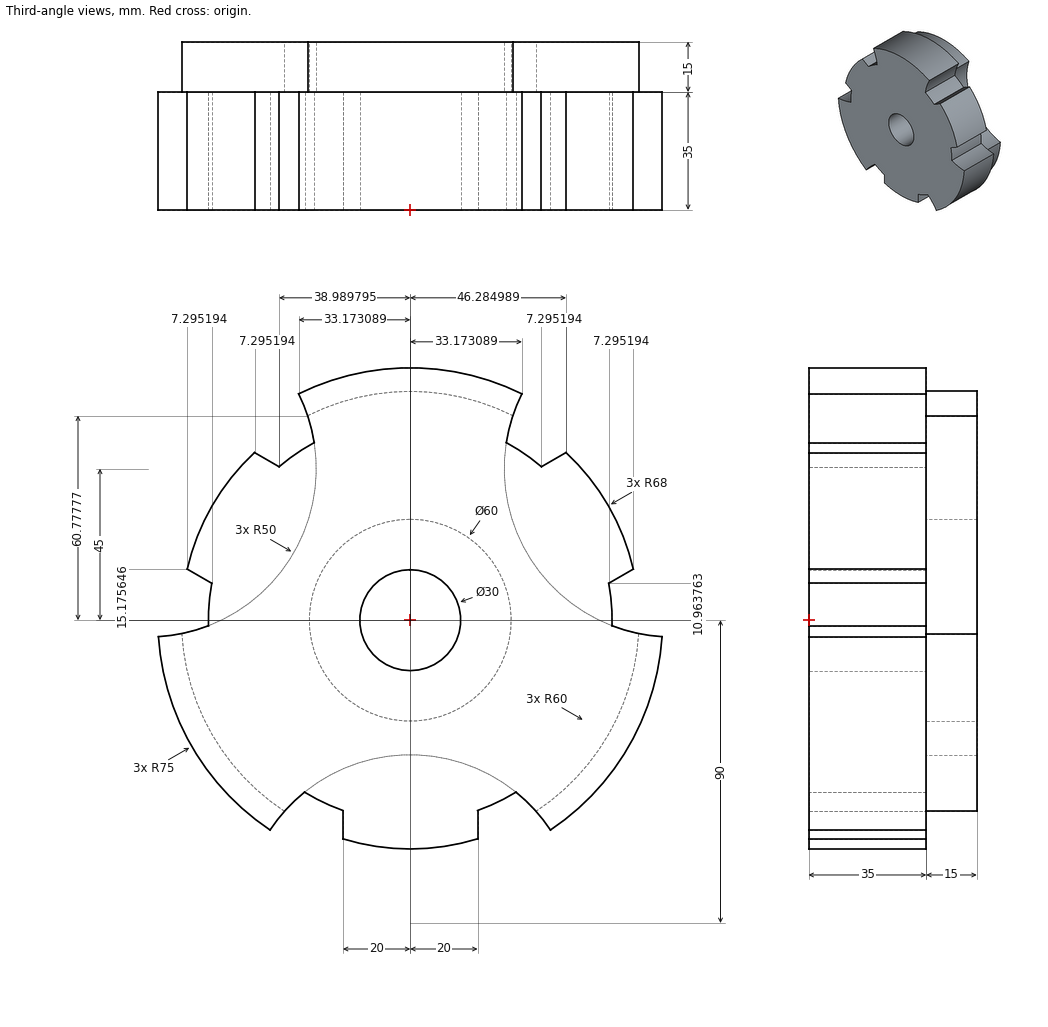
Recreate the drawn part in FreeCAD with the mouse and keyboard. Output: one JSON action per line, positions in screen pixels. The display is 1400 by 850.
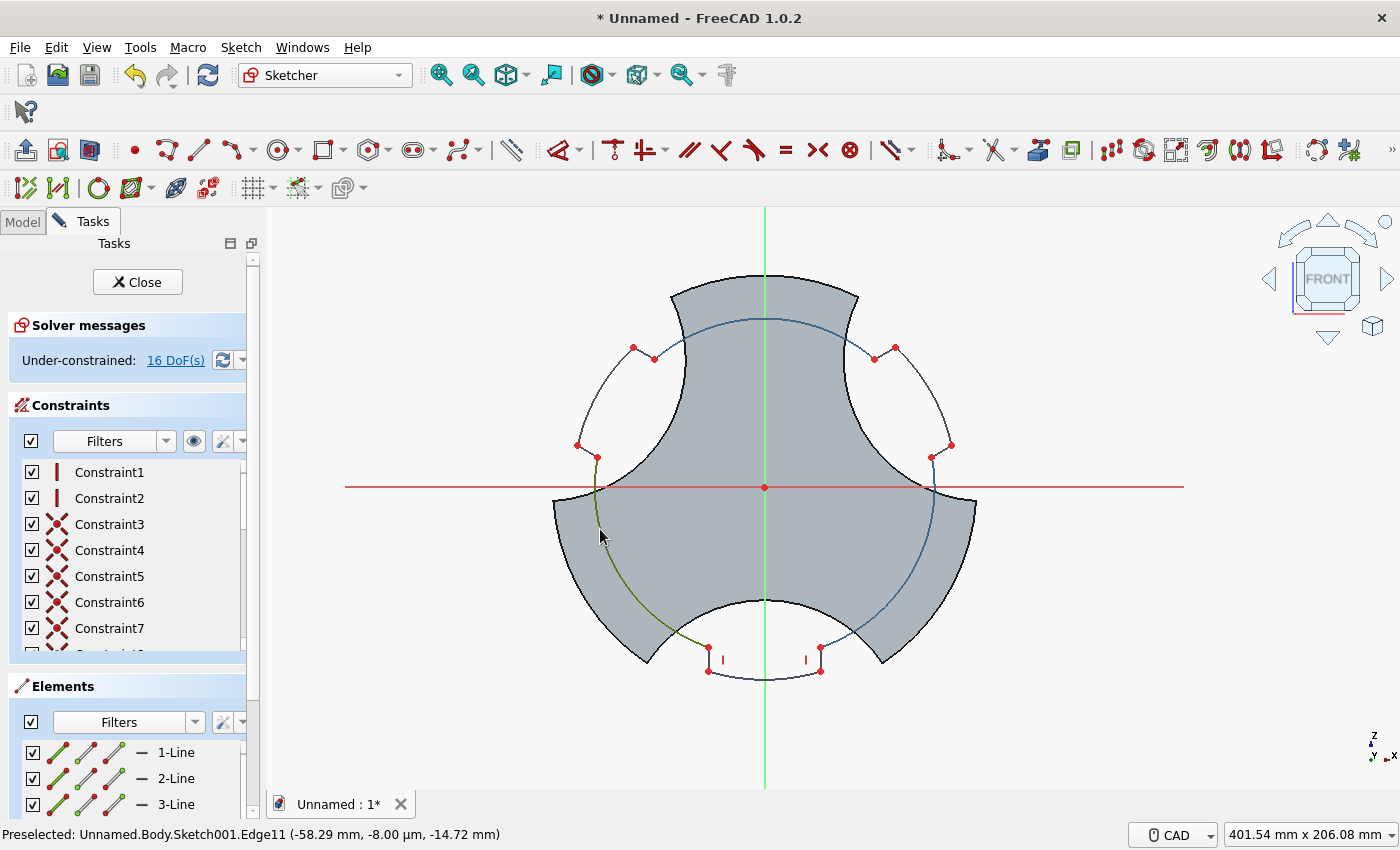
{"action": "key", "text": "e"}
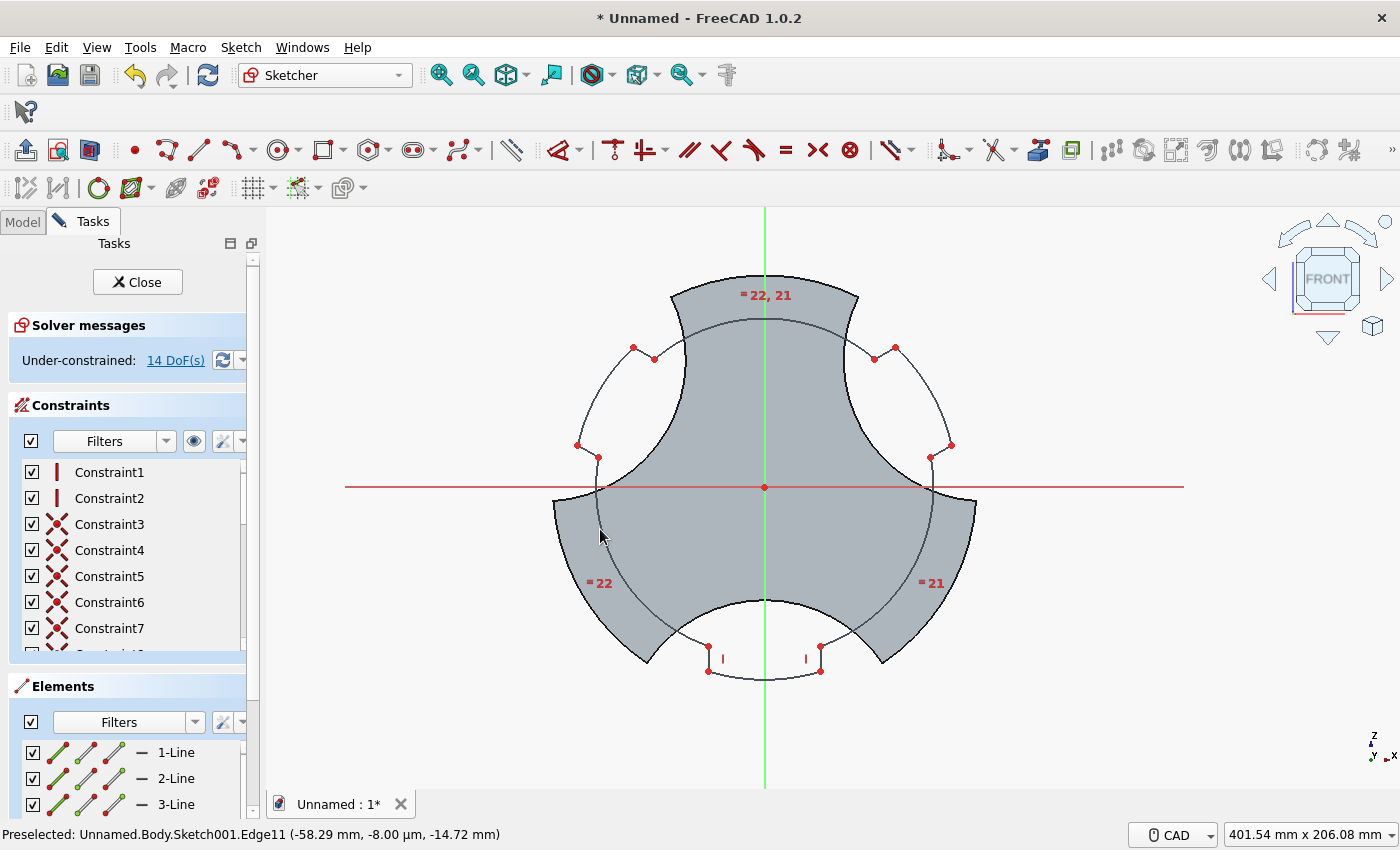
{"action": "left_click", "coordinate": [941, 413]}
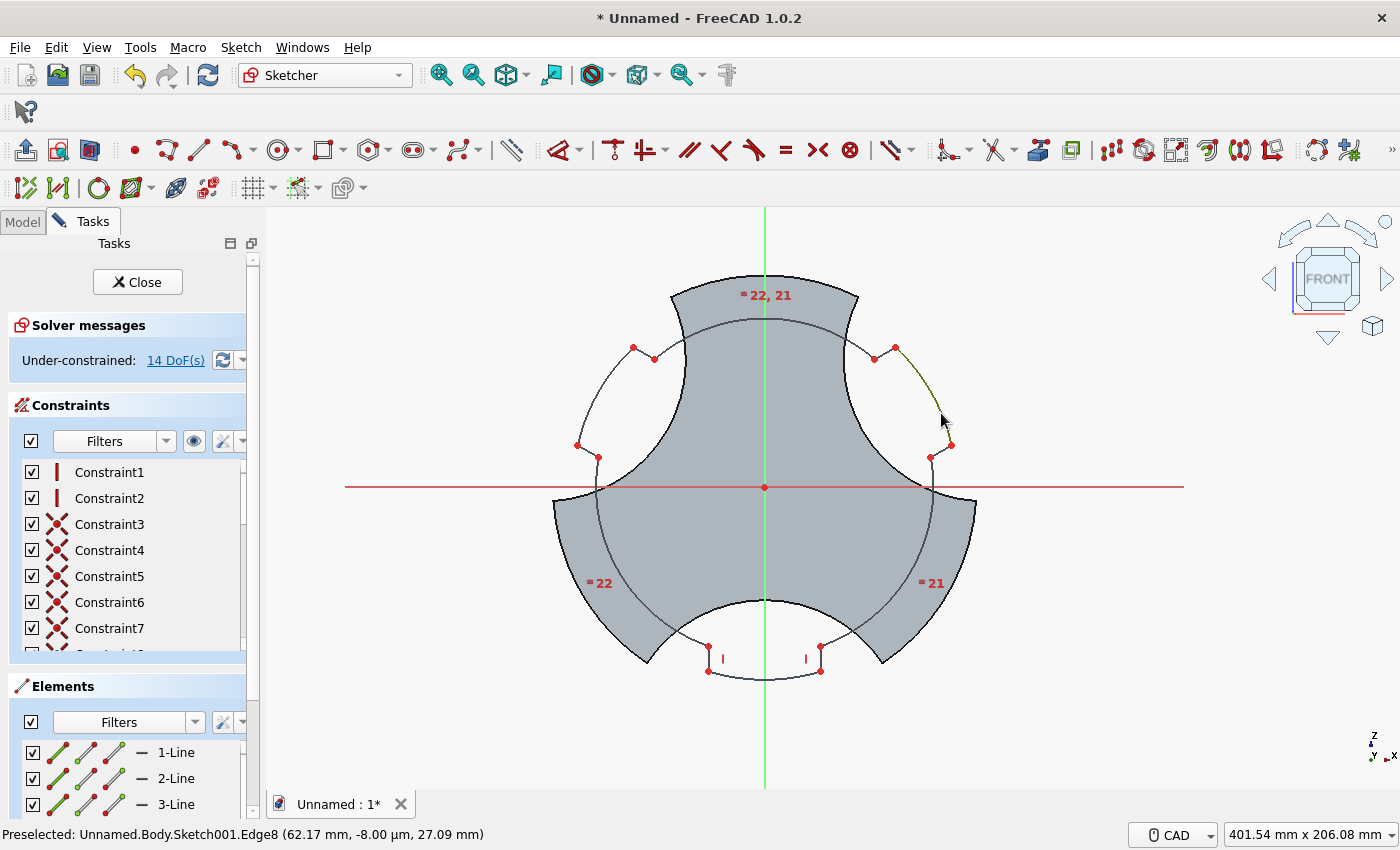
{"action": "left_click", "coordinate": [611, 373]}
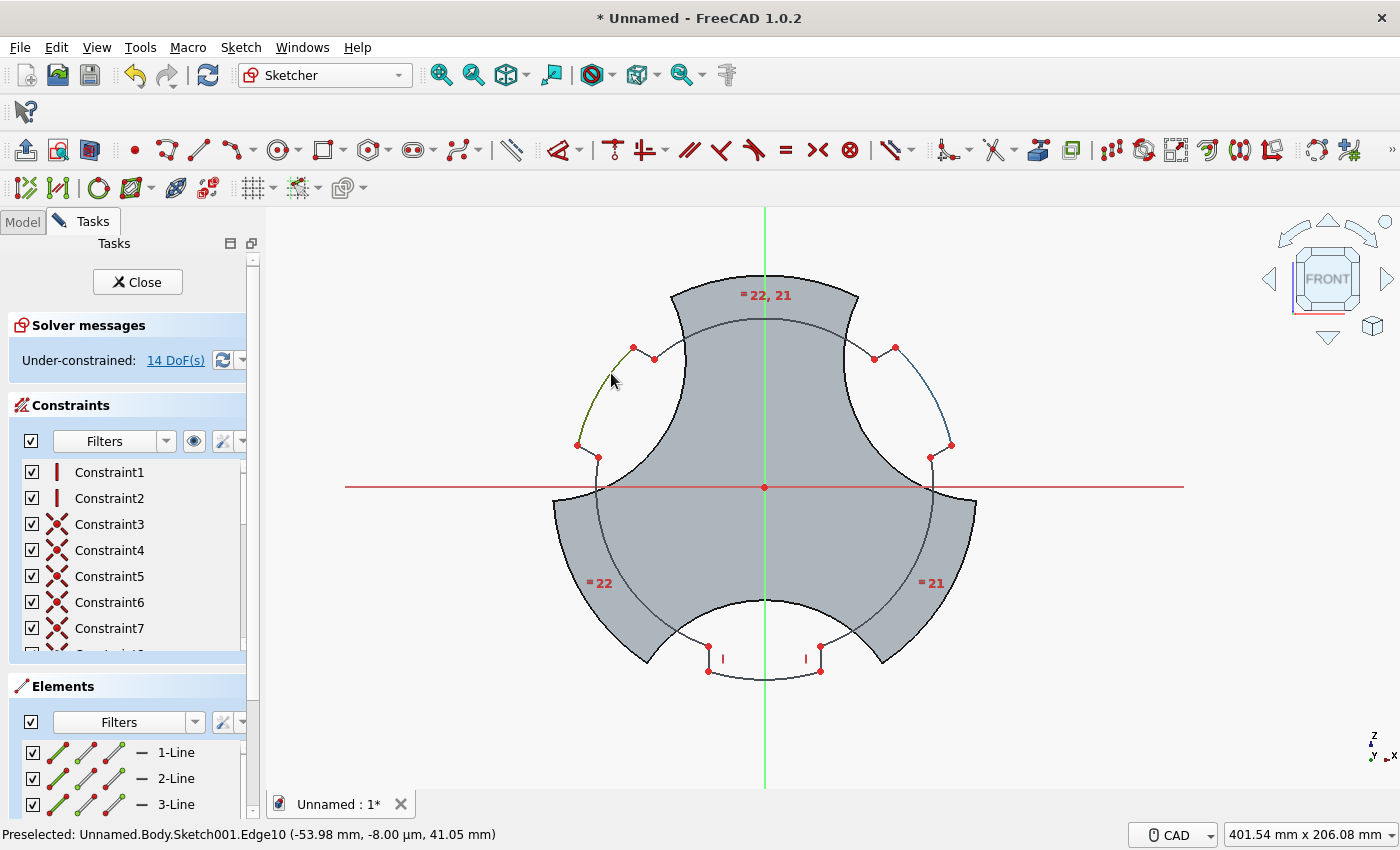
{"action": "left_click", "coordinate": [742, 678]}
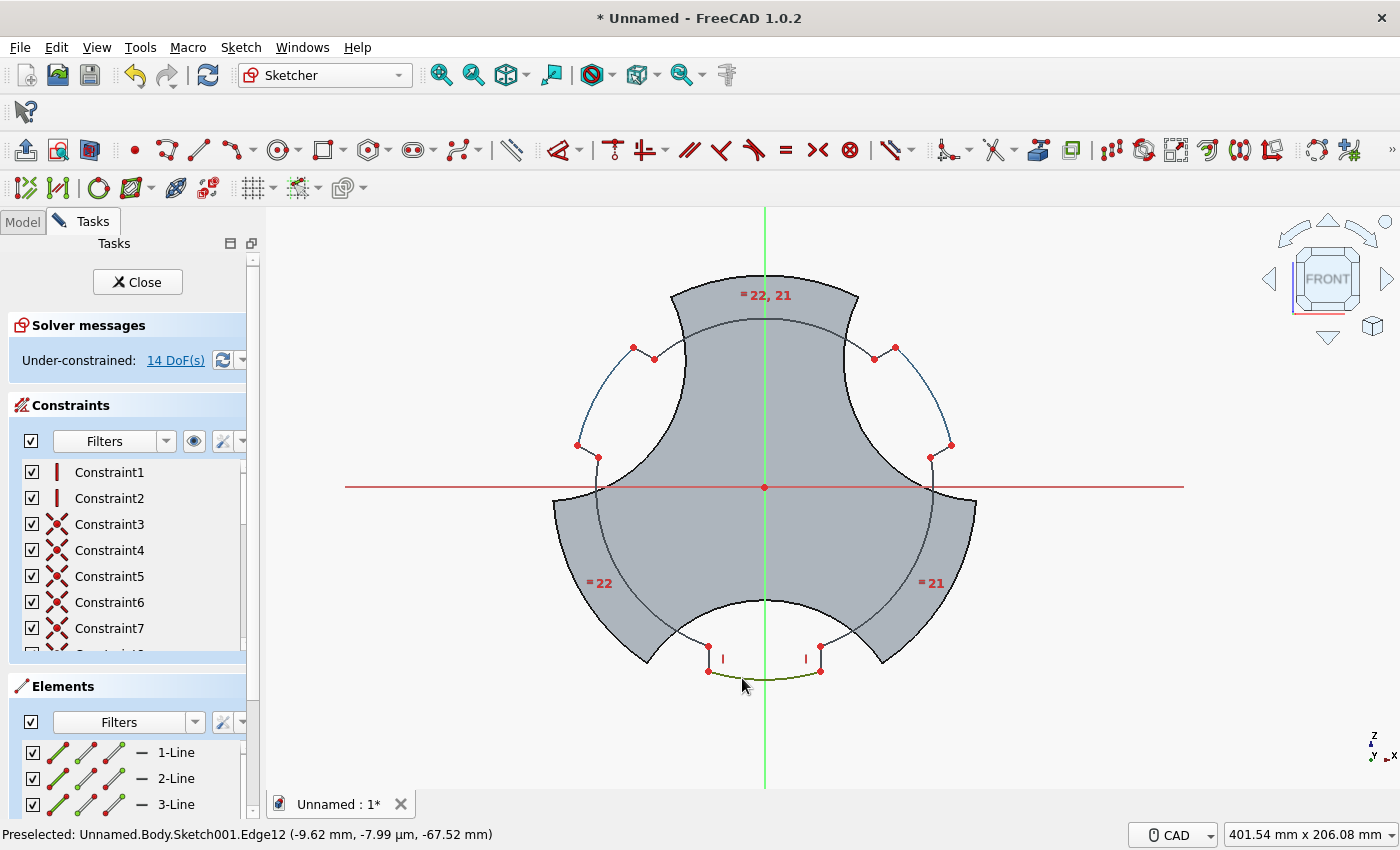
{"action": "left_click", "coordinate": [786, 150]}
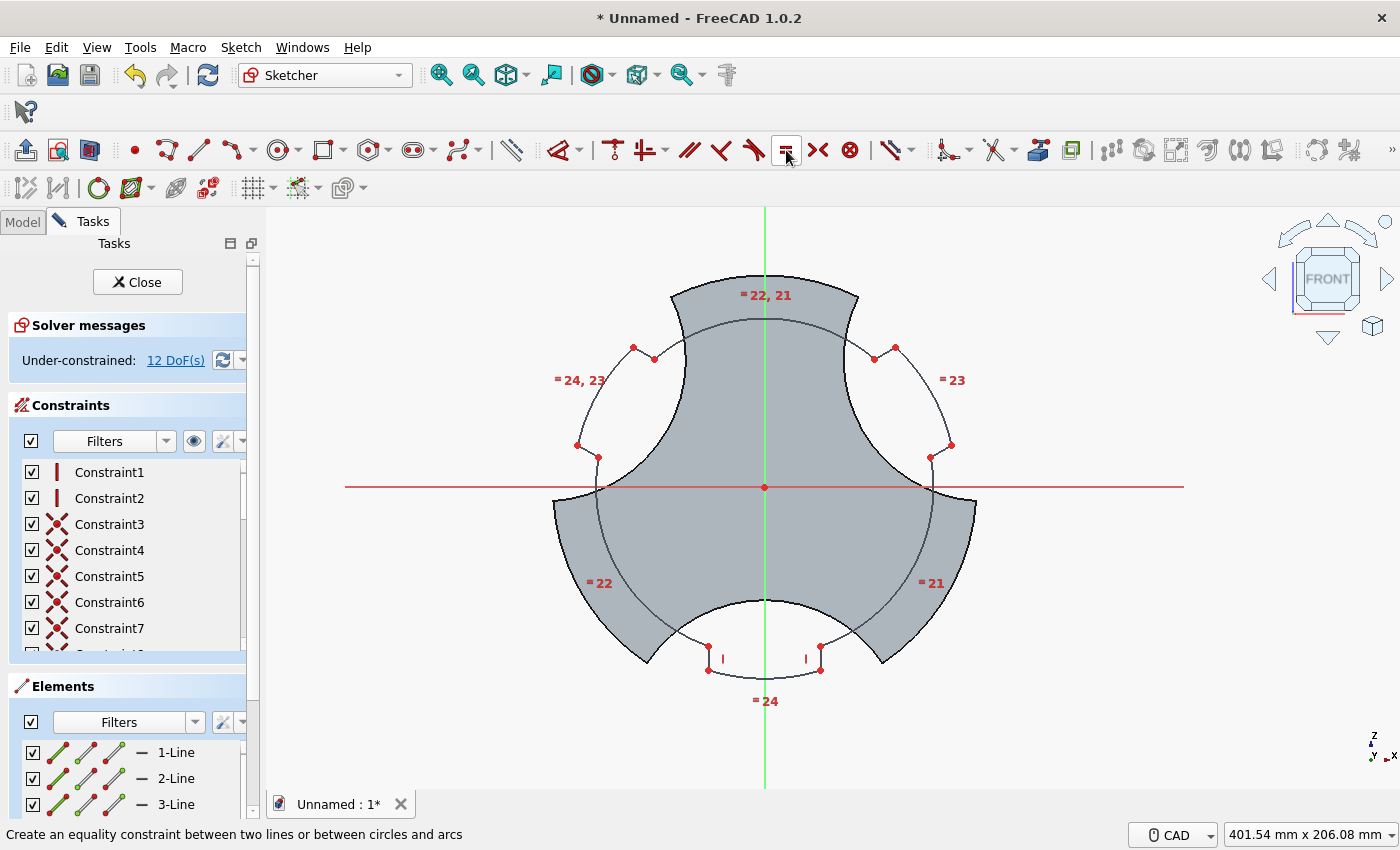
{"action": "left_click", "coordinate": [558, 150]}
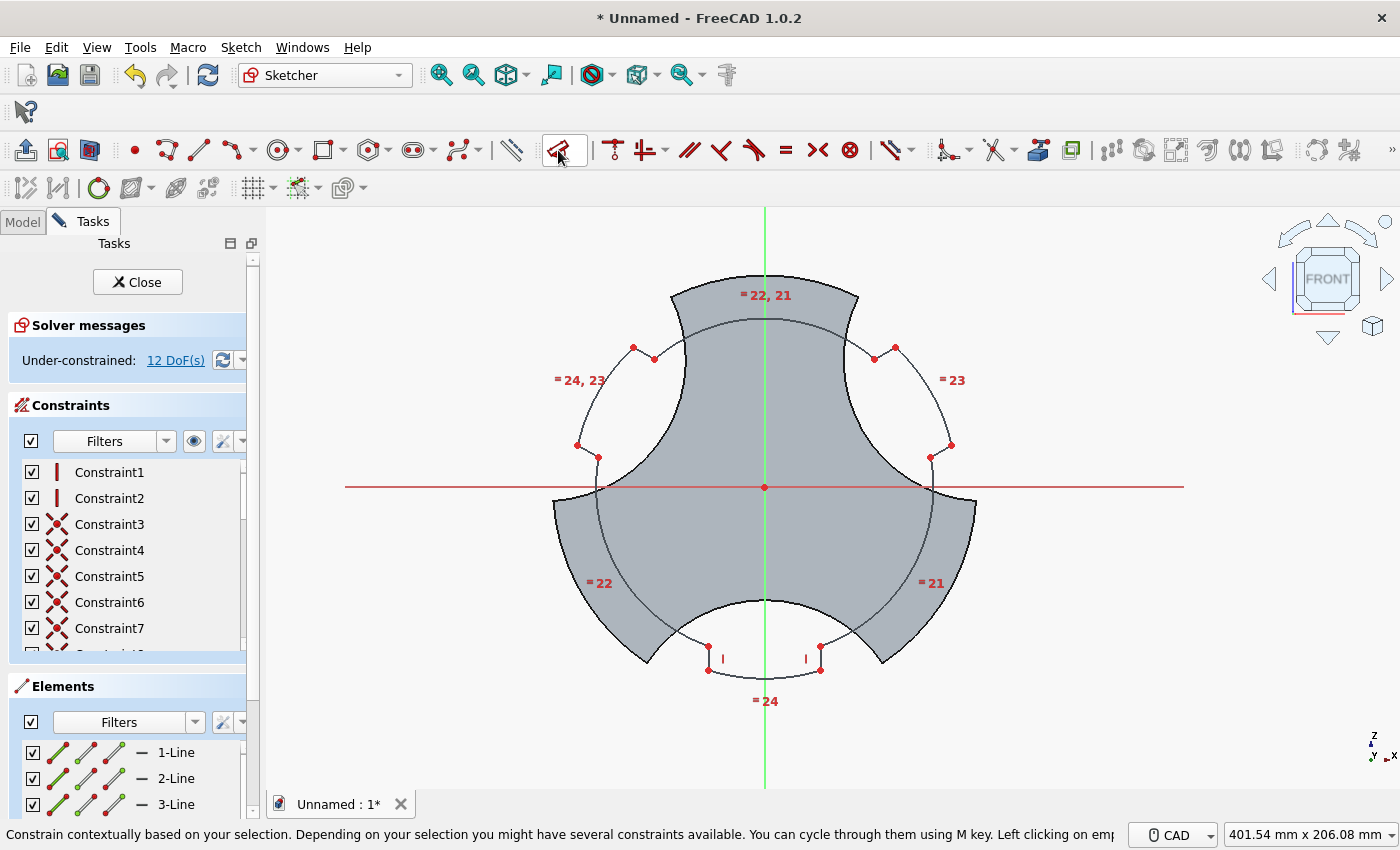
{"action": "left_click", "coordinate": [881, 609]}
{"action": "left_click", "coordinate": [903, 632]}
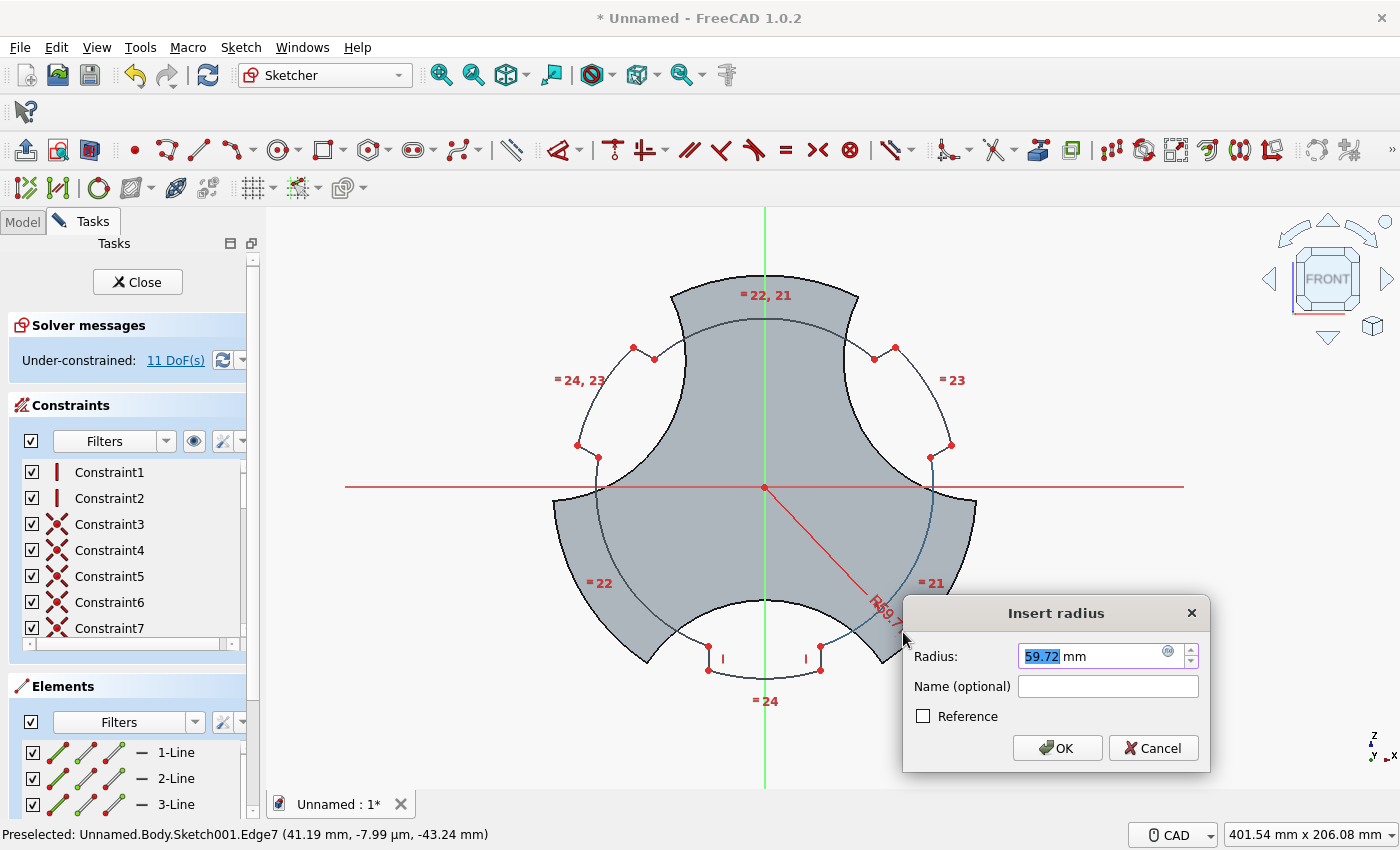
{"action": "type", "text": "60"}
{"action": "key", "text": "Return"}